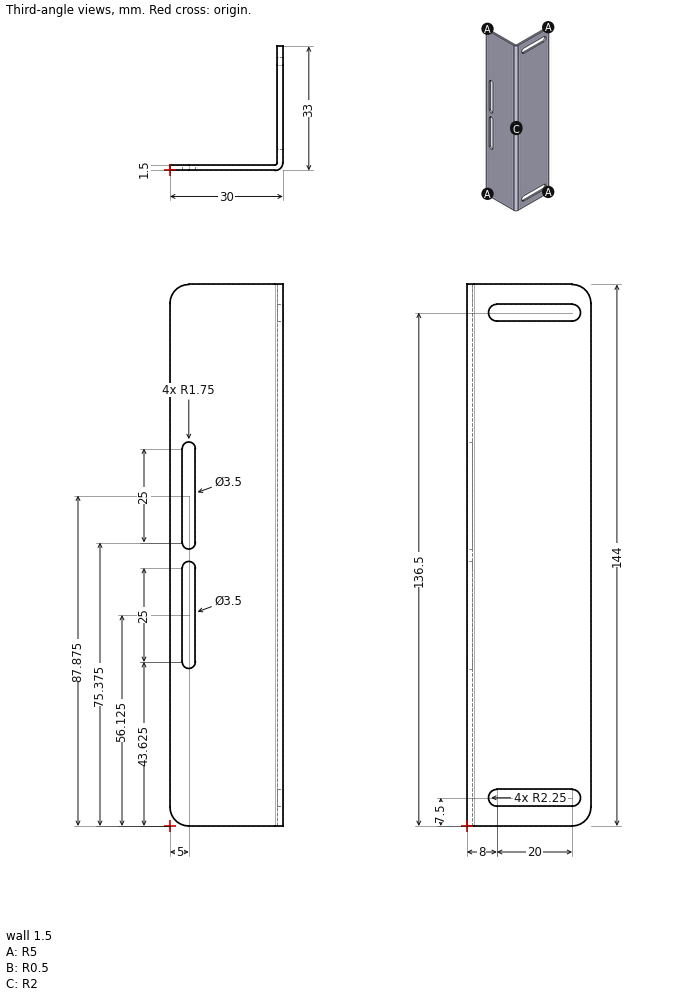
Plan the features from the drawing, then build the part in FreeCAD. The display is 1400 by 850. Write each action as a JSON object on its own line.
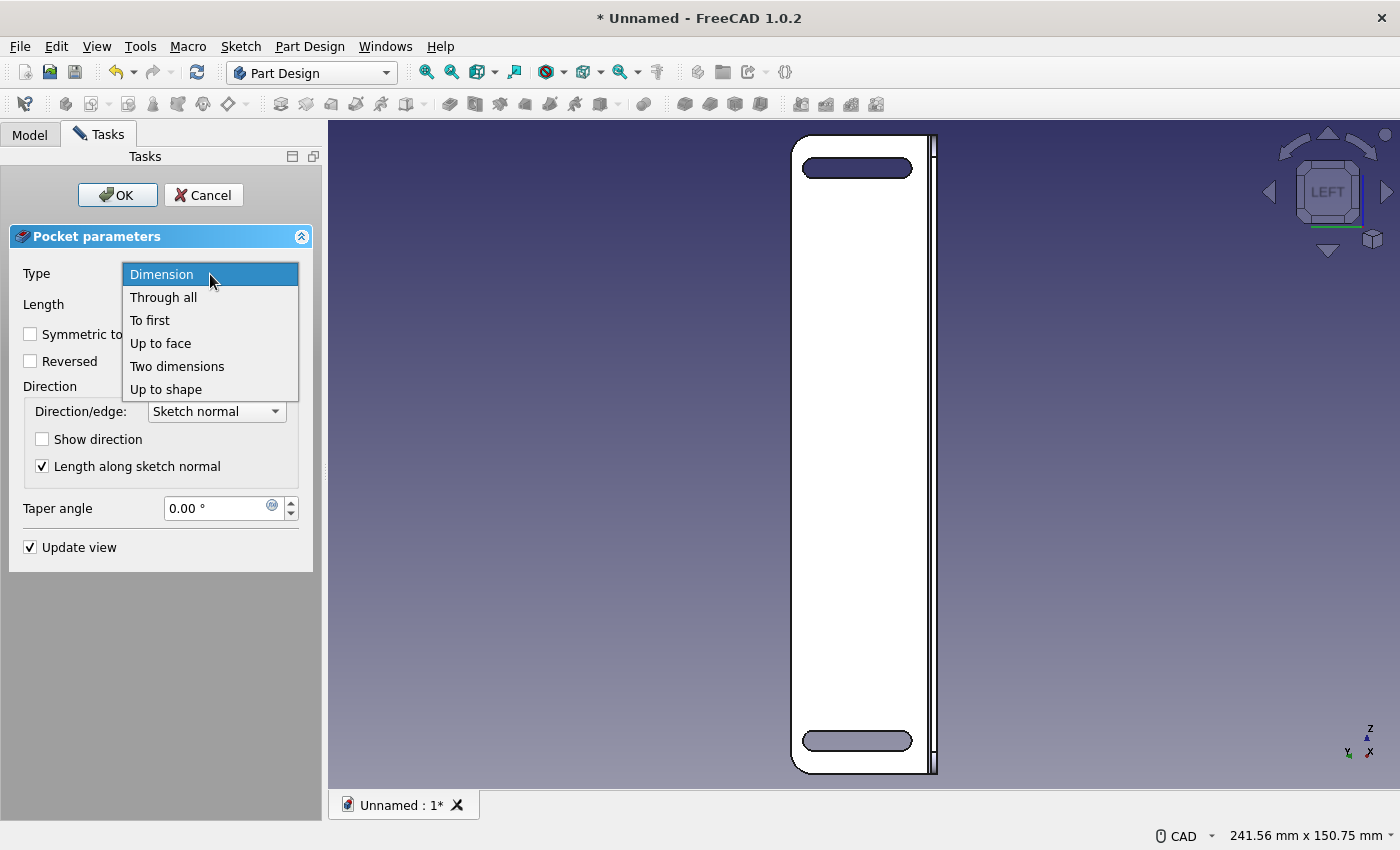
{"action": "left_click", "coordinate": [208, 298]}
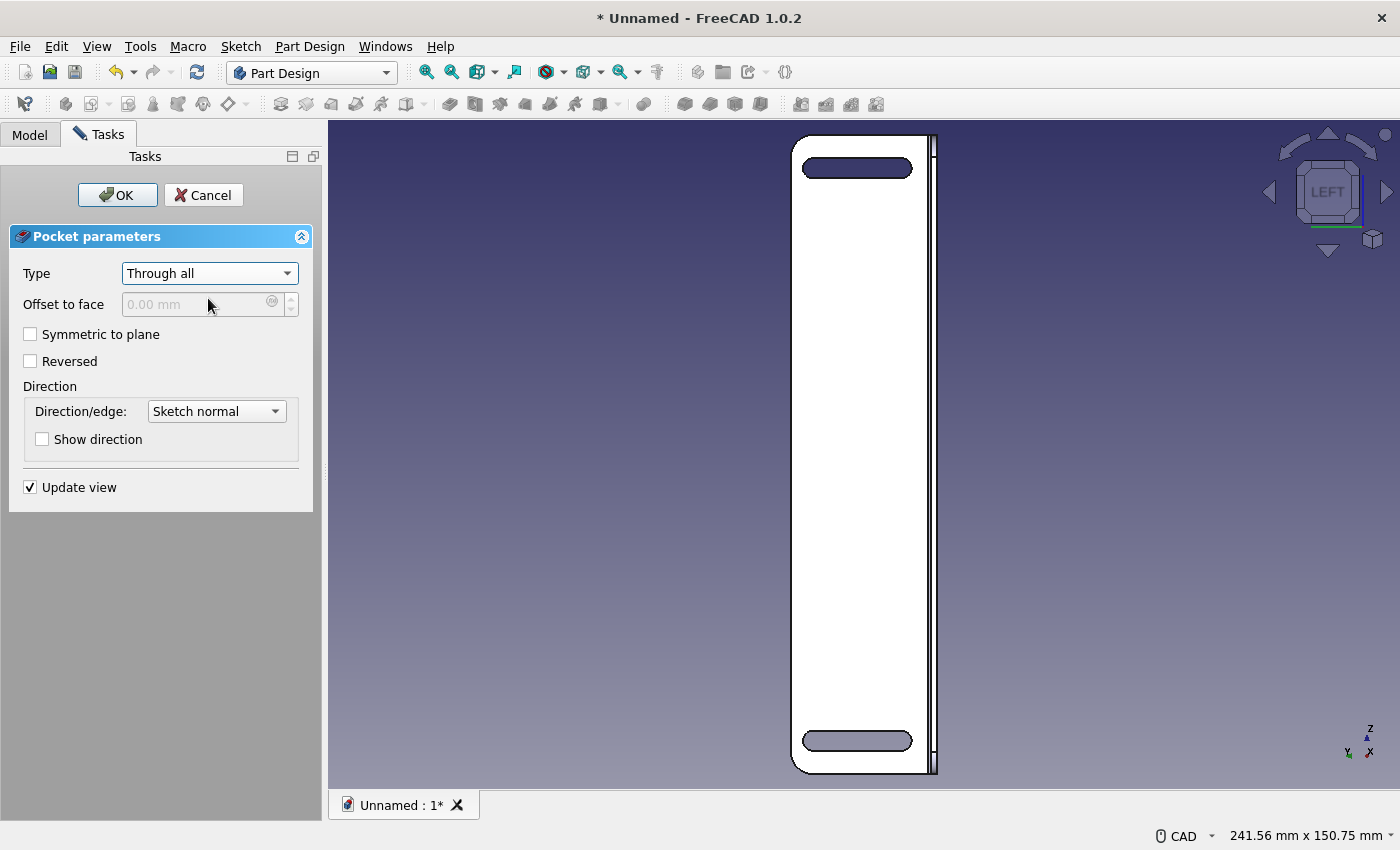
{"action": "left_click", "coordinate": [118, 195]}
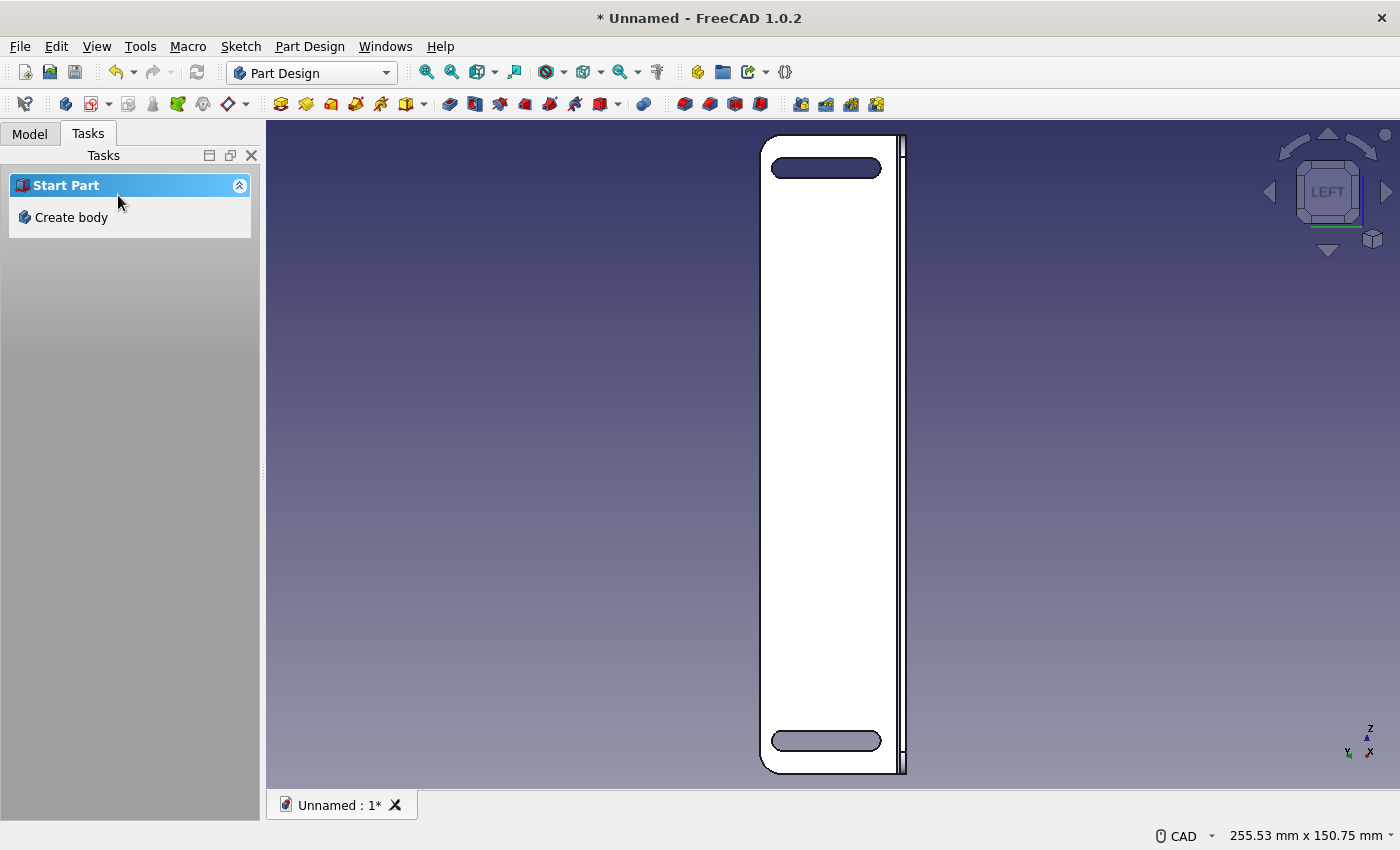
{"action": "left_click", "coordinate": [90, 104]}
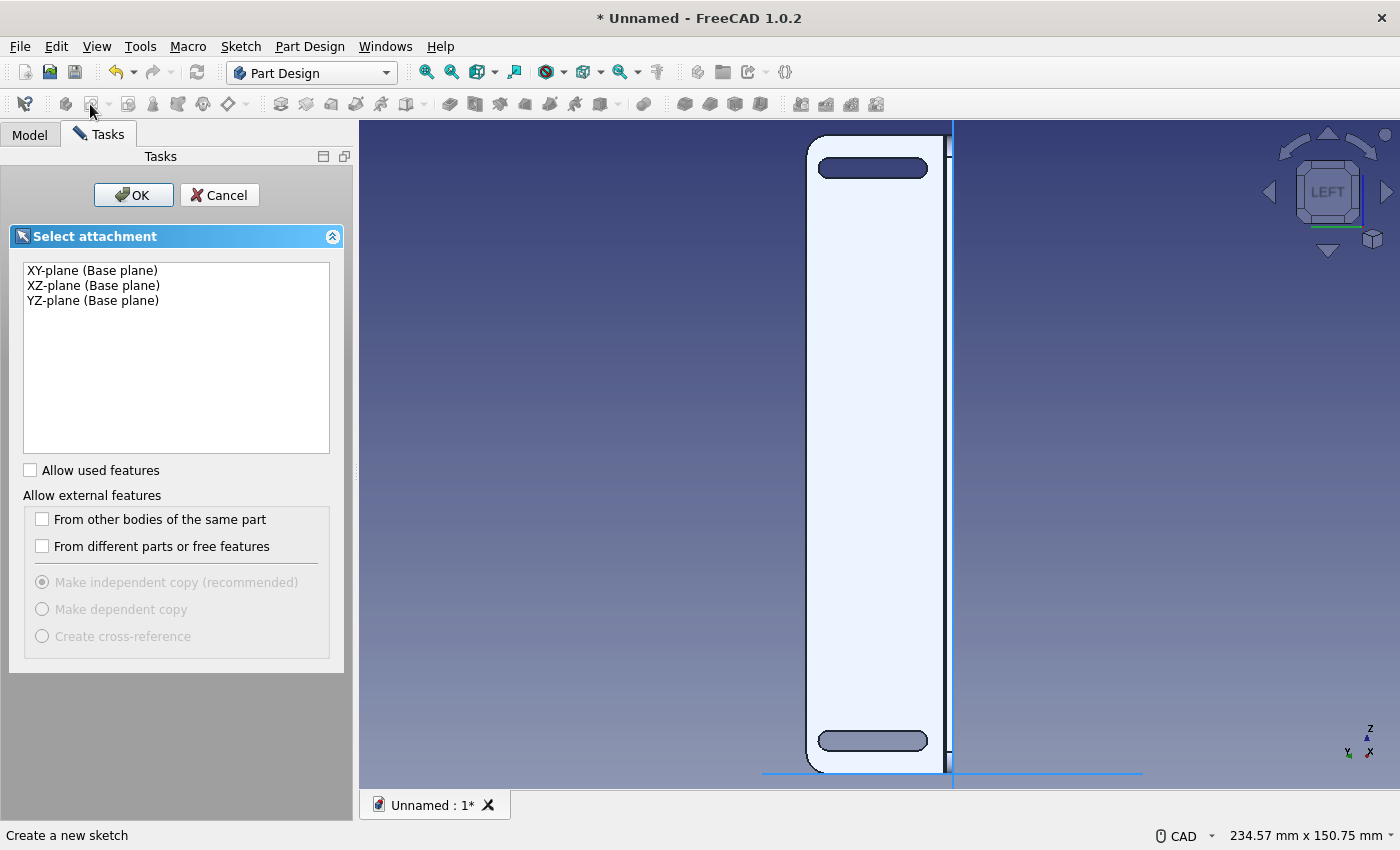
{"action": "left_click", "coordinate": [84, 286]}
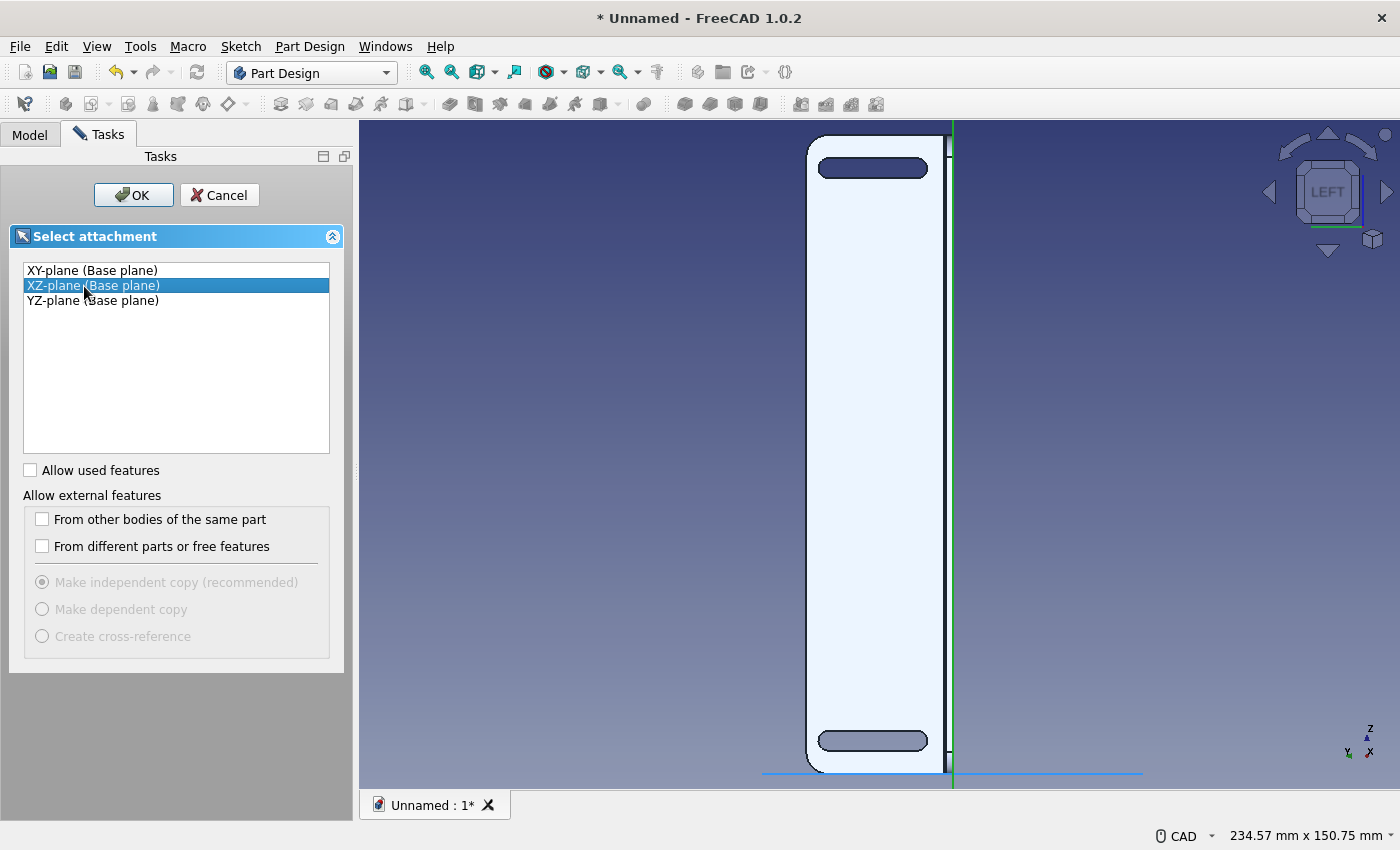
{"action": "left_click", "coordinate": [134, 195]}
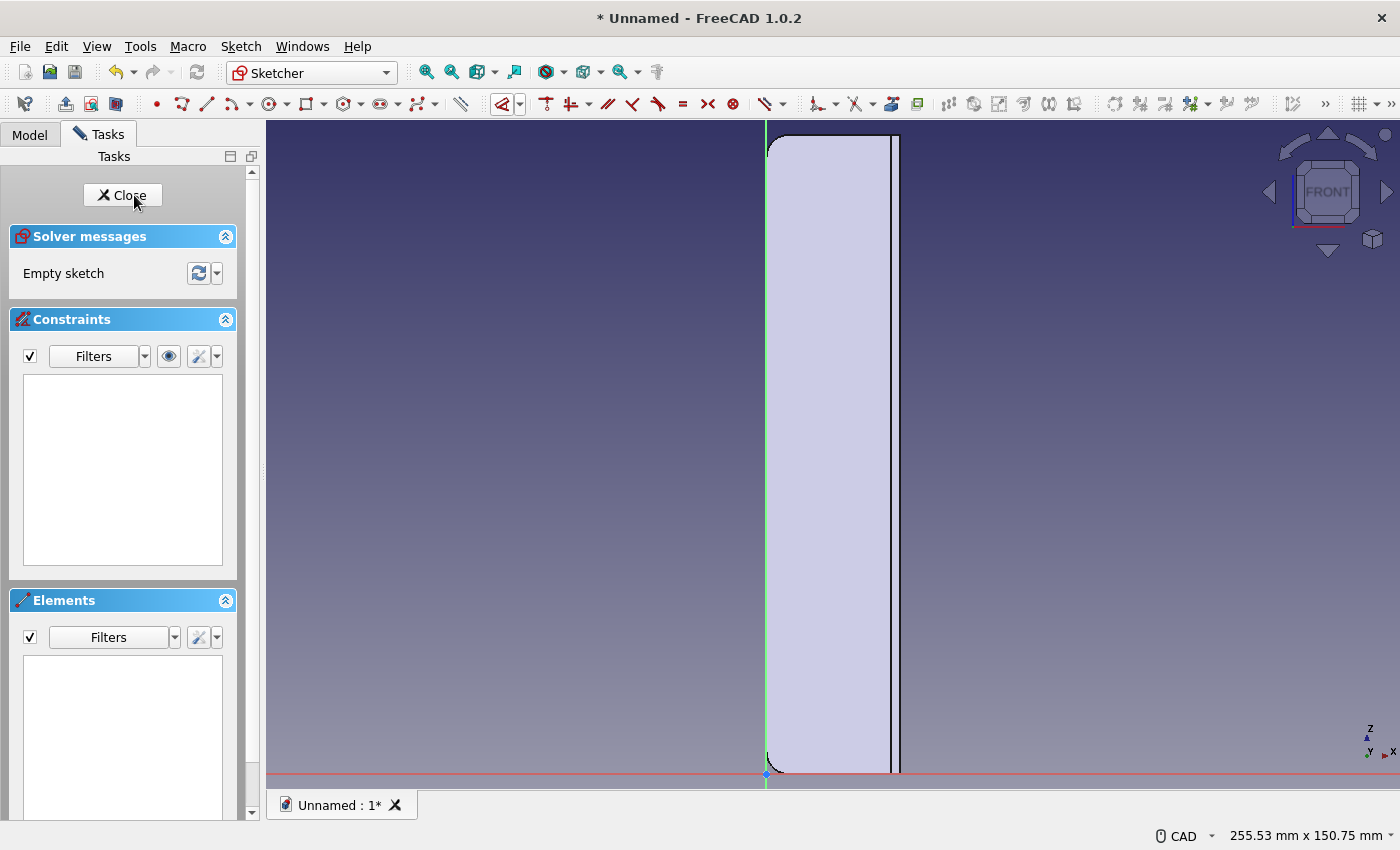
{"action": "scroll", "coordinate": [790, 380], "scroll_direction": "up", "scroll_amount": 15}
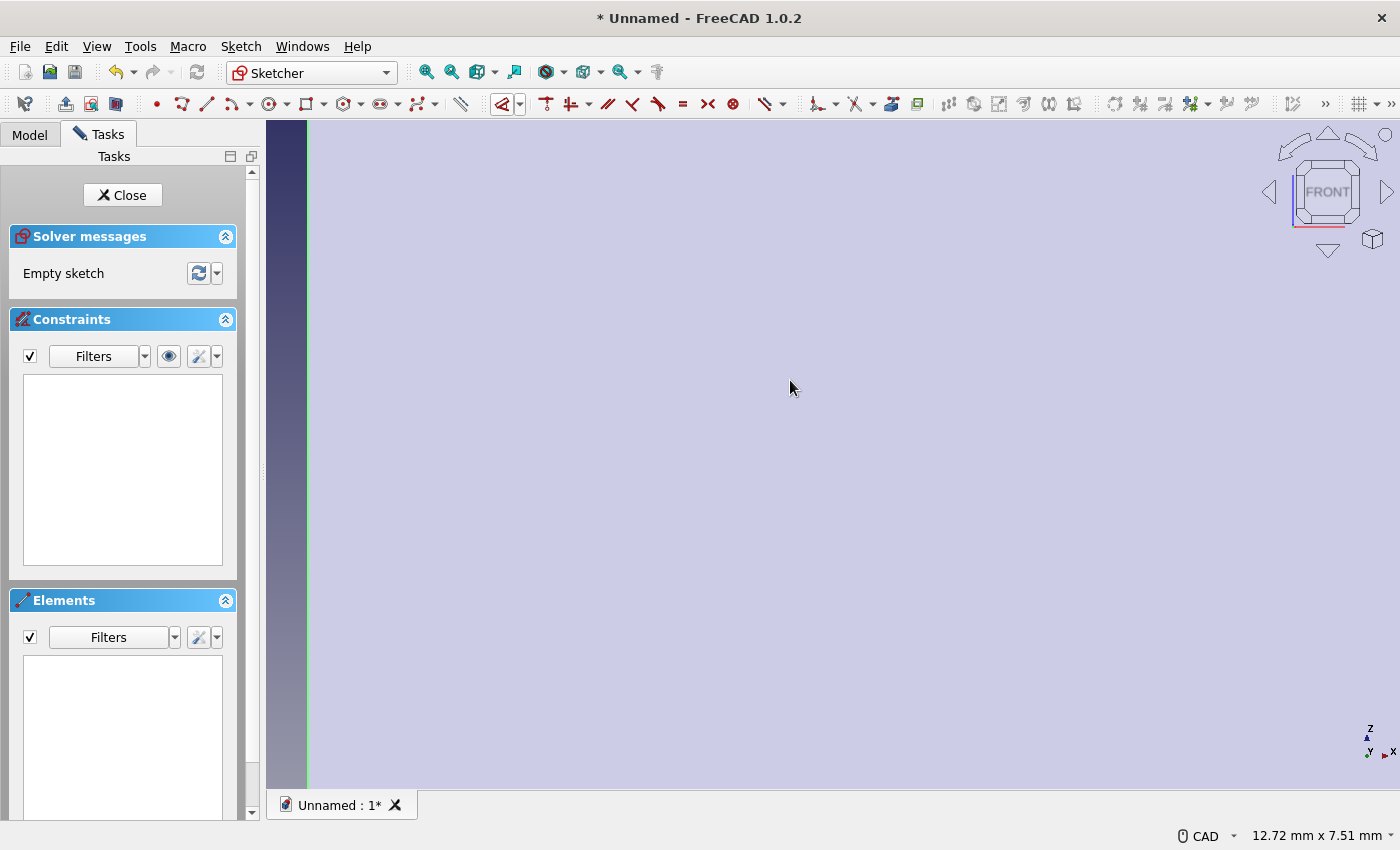
{"action": "scroll", "coordinate": [731, 453], "scroll_direction": "up", "scroll_amount": 2}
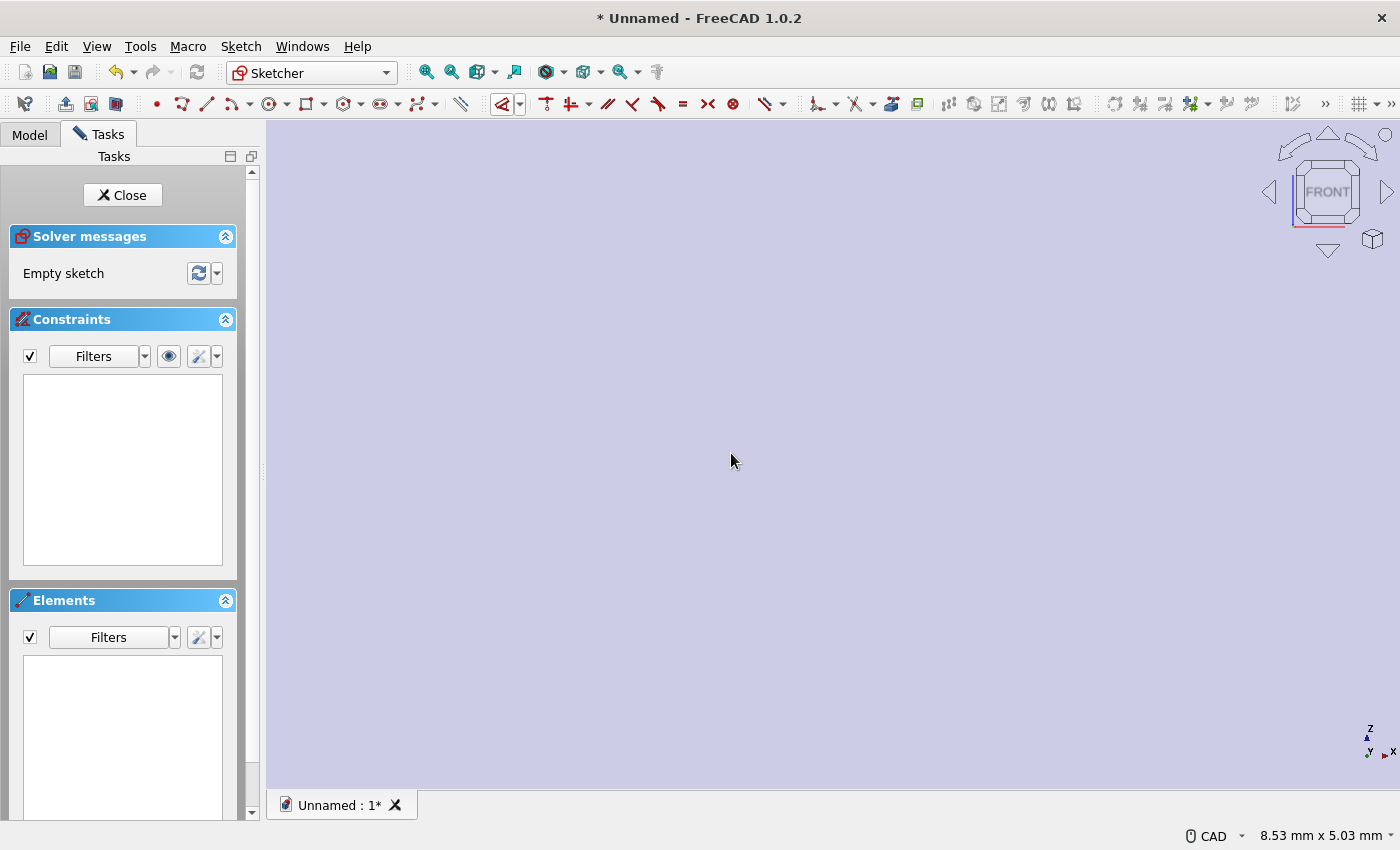
{"action": "left_click", "coordinate": [268, 104]}